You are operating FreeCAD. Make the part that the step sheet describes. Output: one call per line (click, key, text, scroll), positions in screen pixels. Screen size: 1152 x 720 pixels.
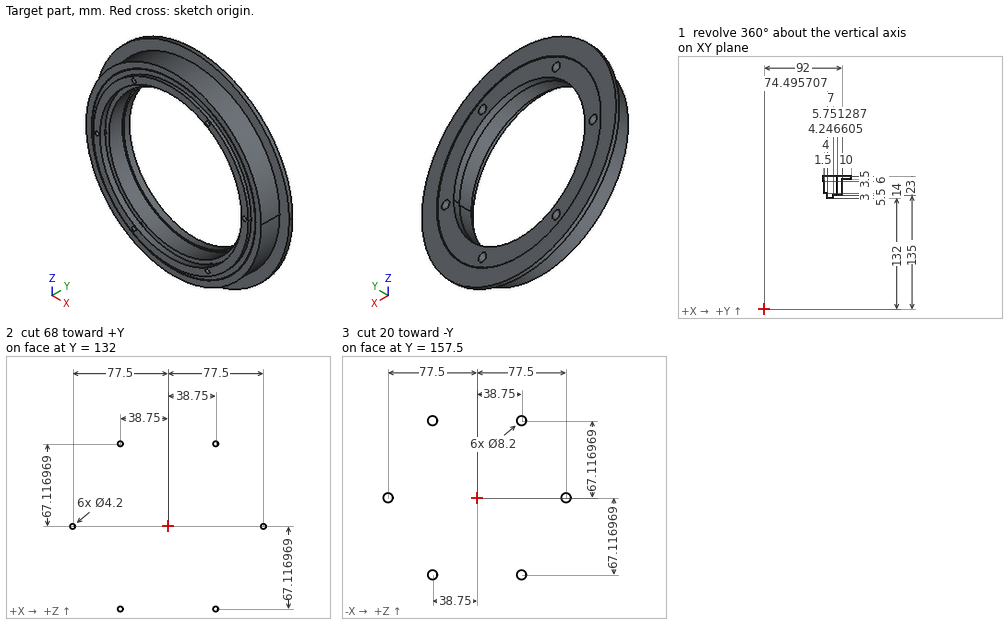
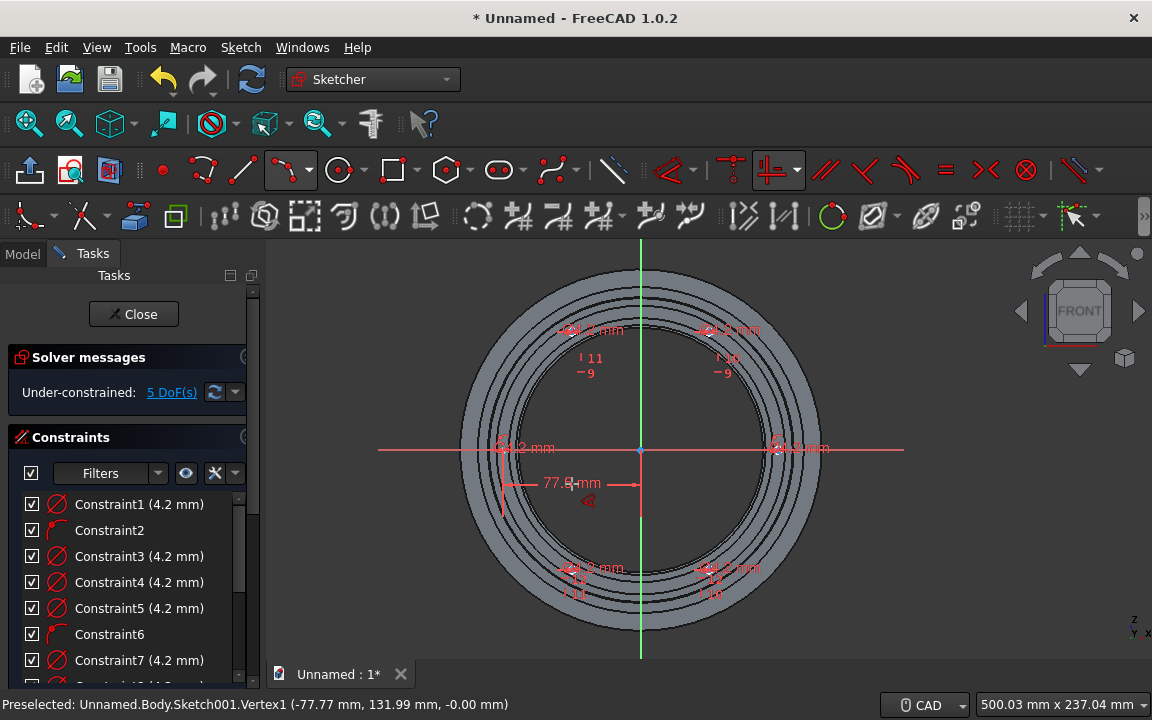
click(778, 450)
click(709, 484)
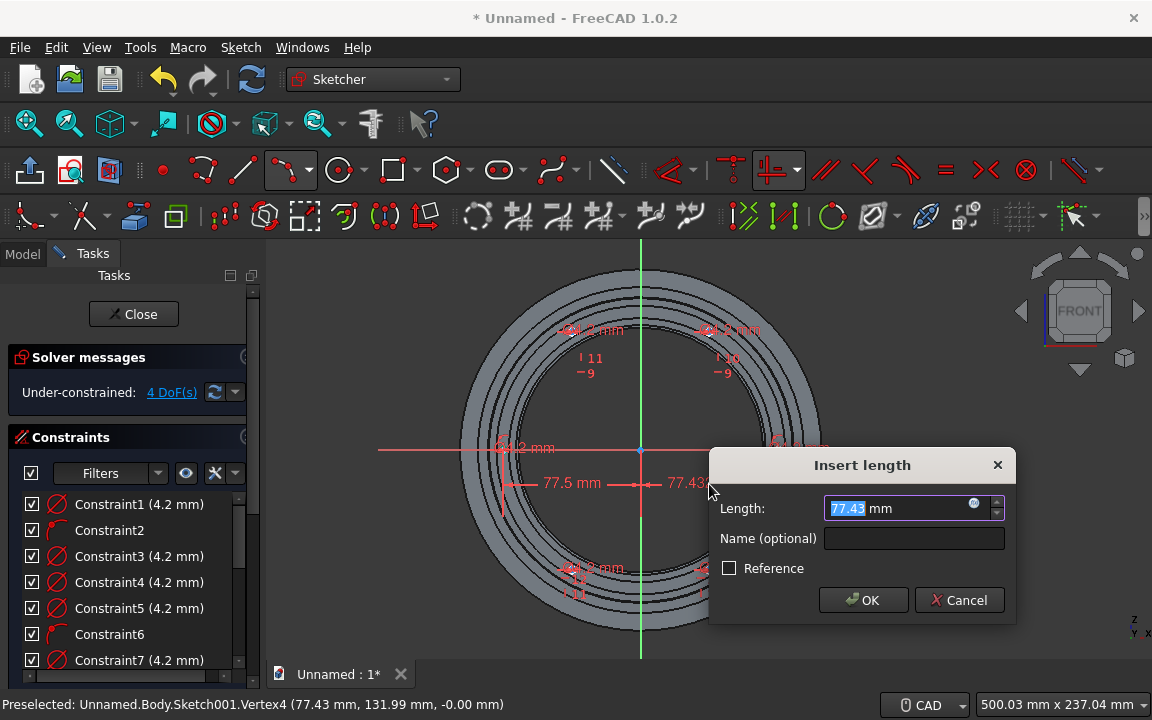
text(77.5)
key(Return)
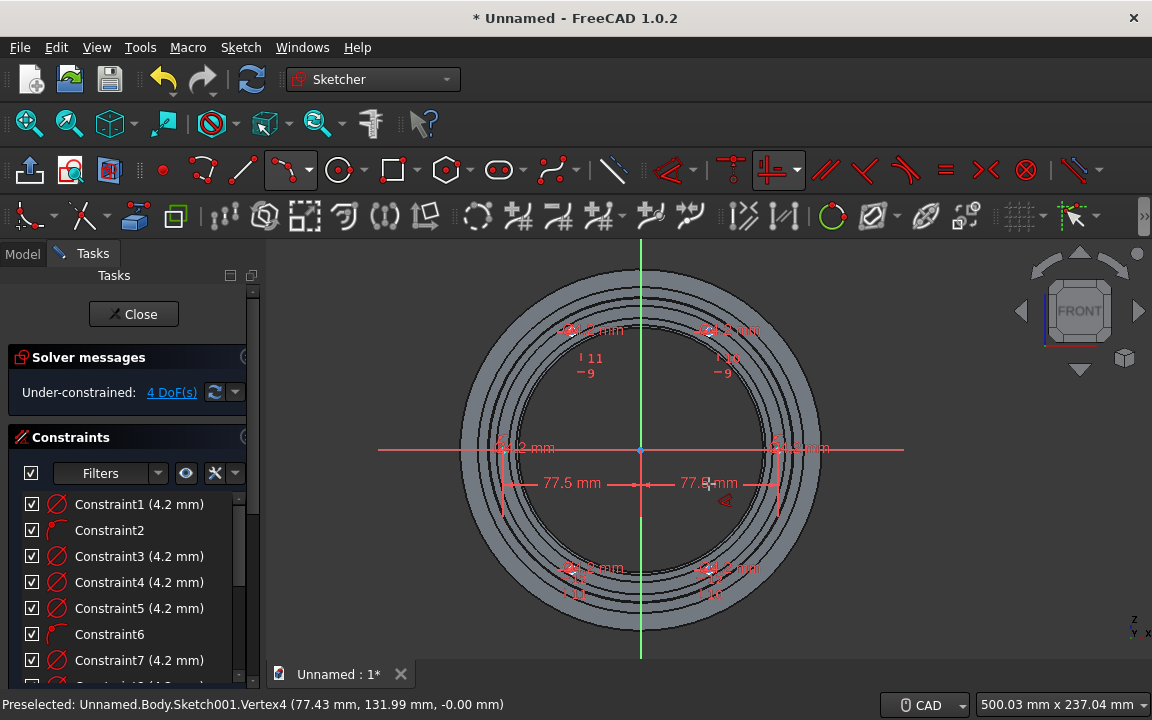
click(572, 332)
click(606, 298)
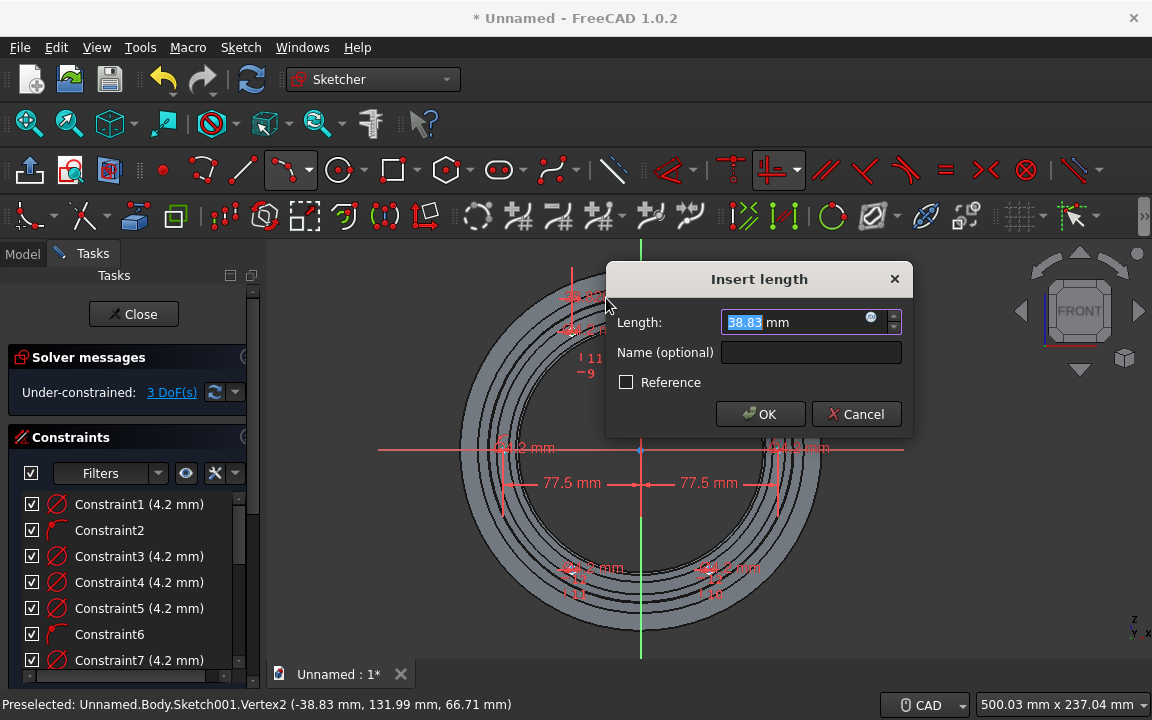
text(38.75)
key(Return)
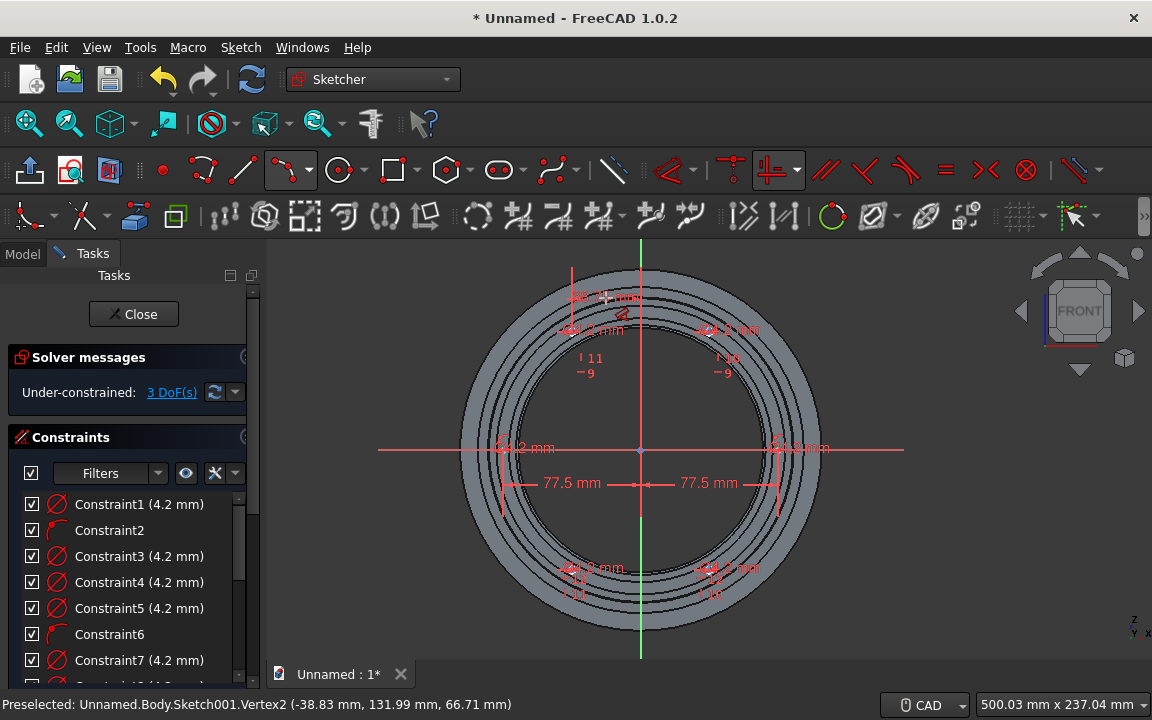
click(709, 332)
click(691, 298)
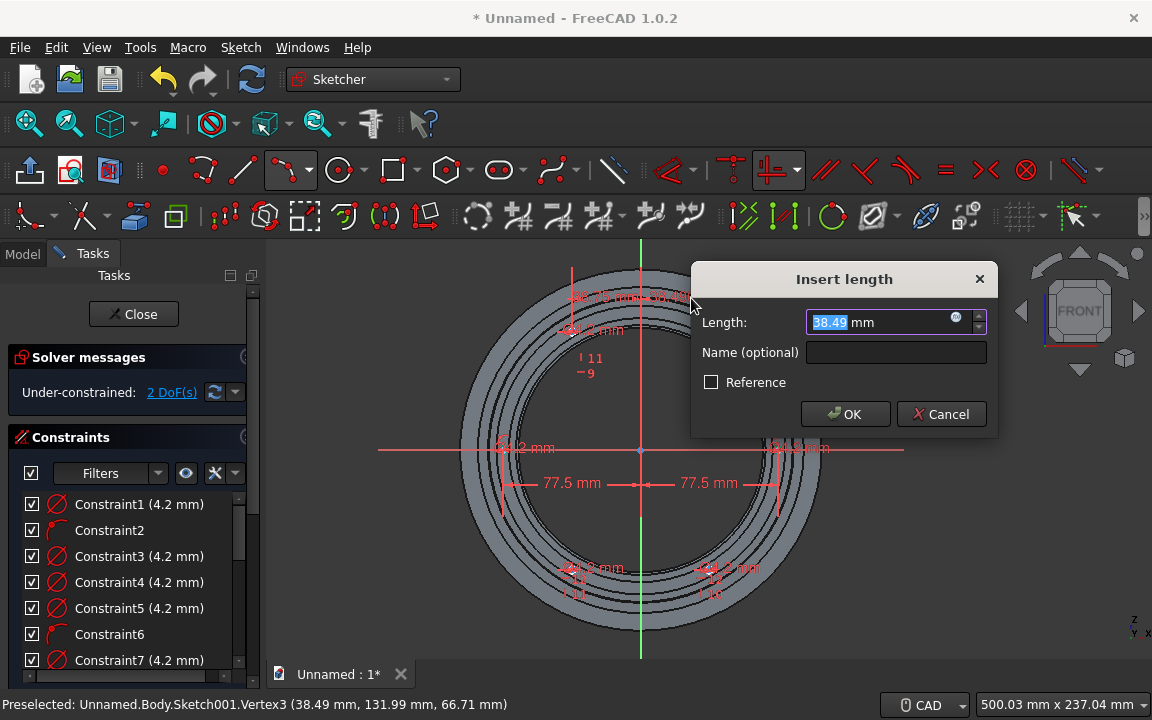
text(38.75)
key(Return)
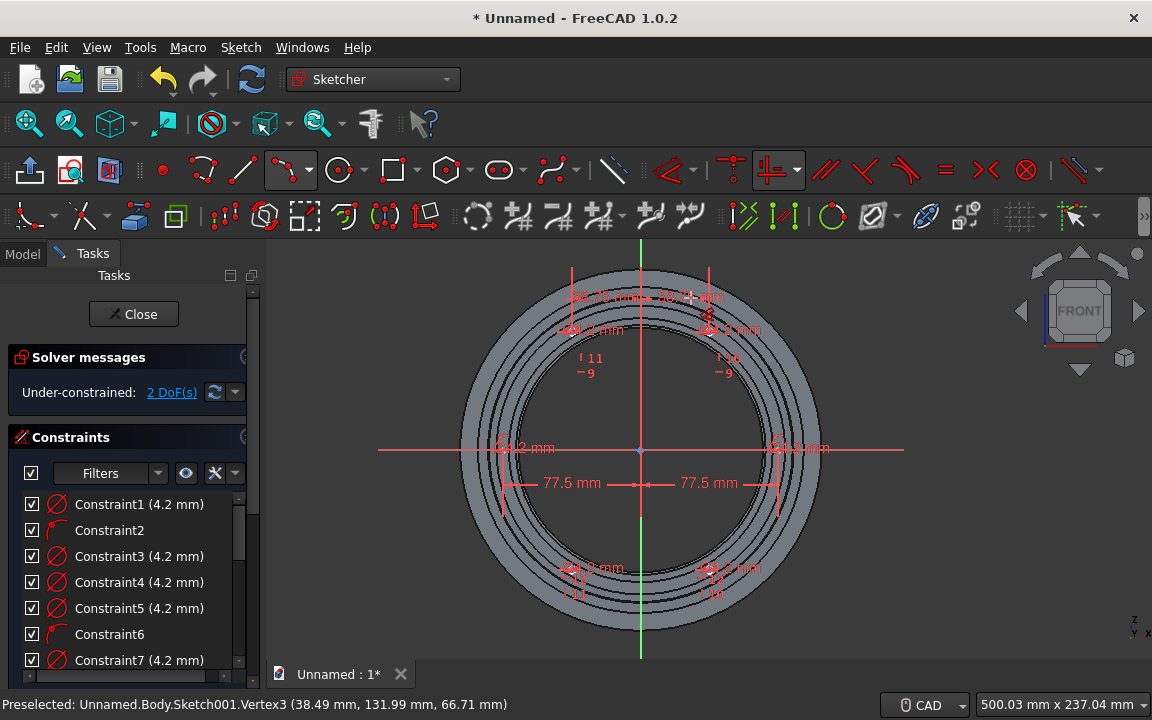
click(572, 332)
click(538, 391)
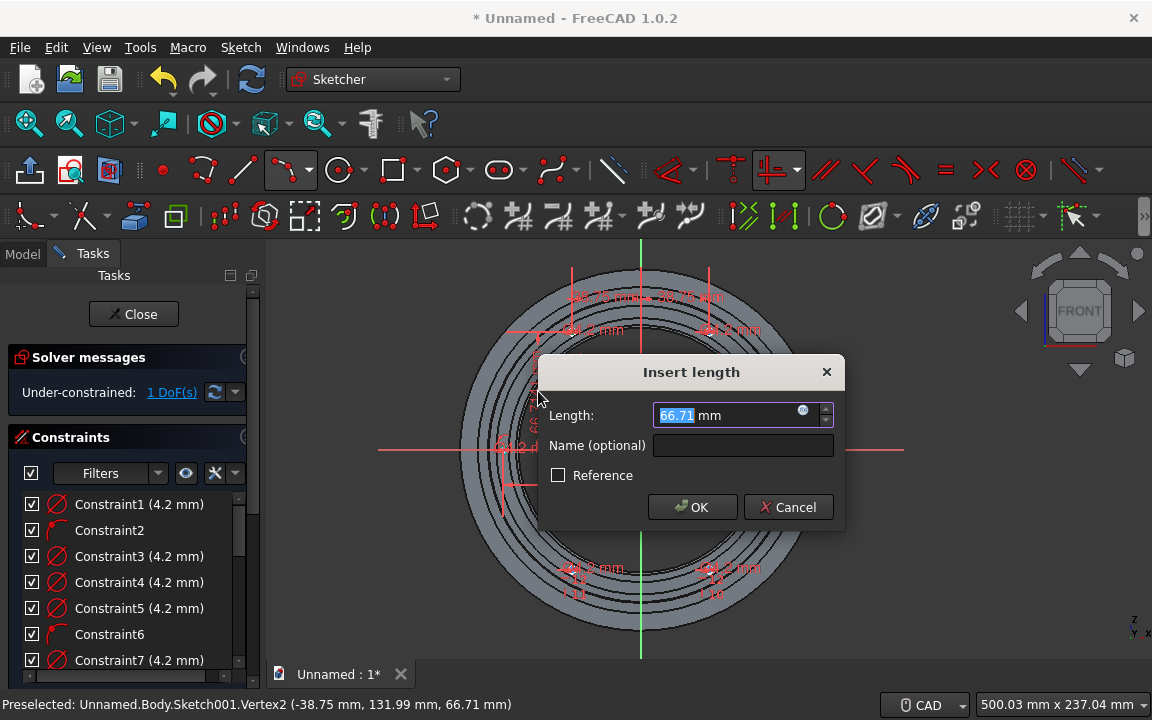
text(67.116969)
key(Return)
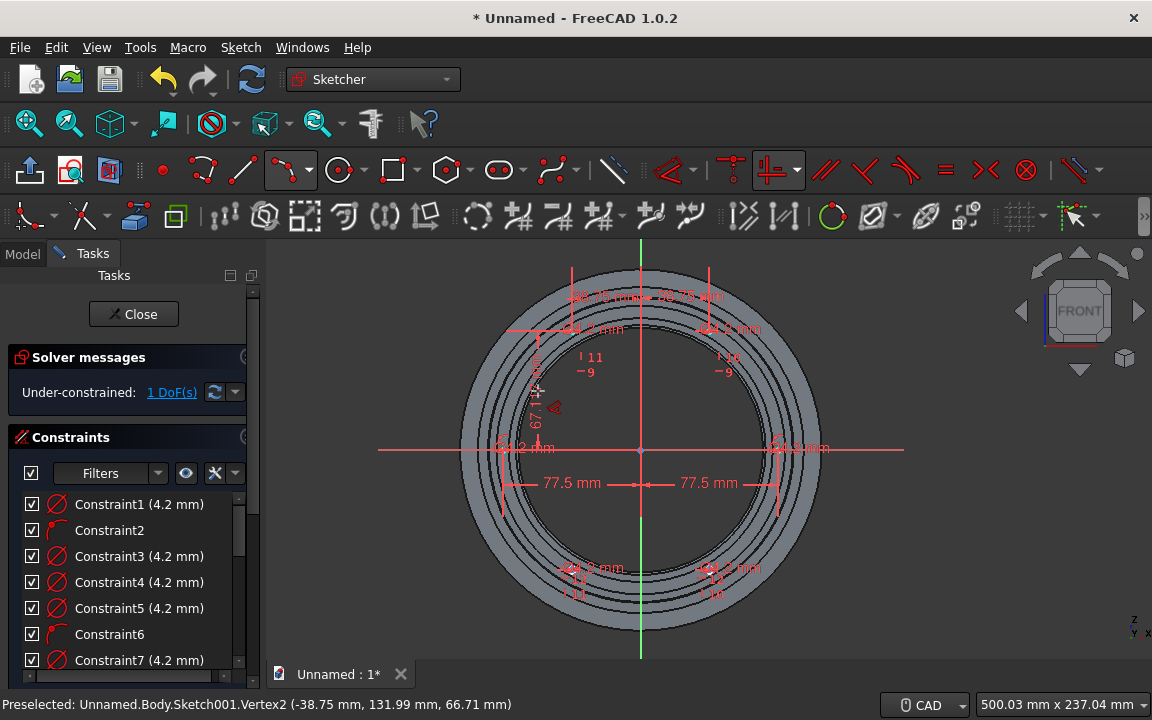
click(709, 570)
click(743, 510)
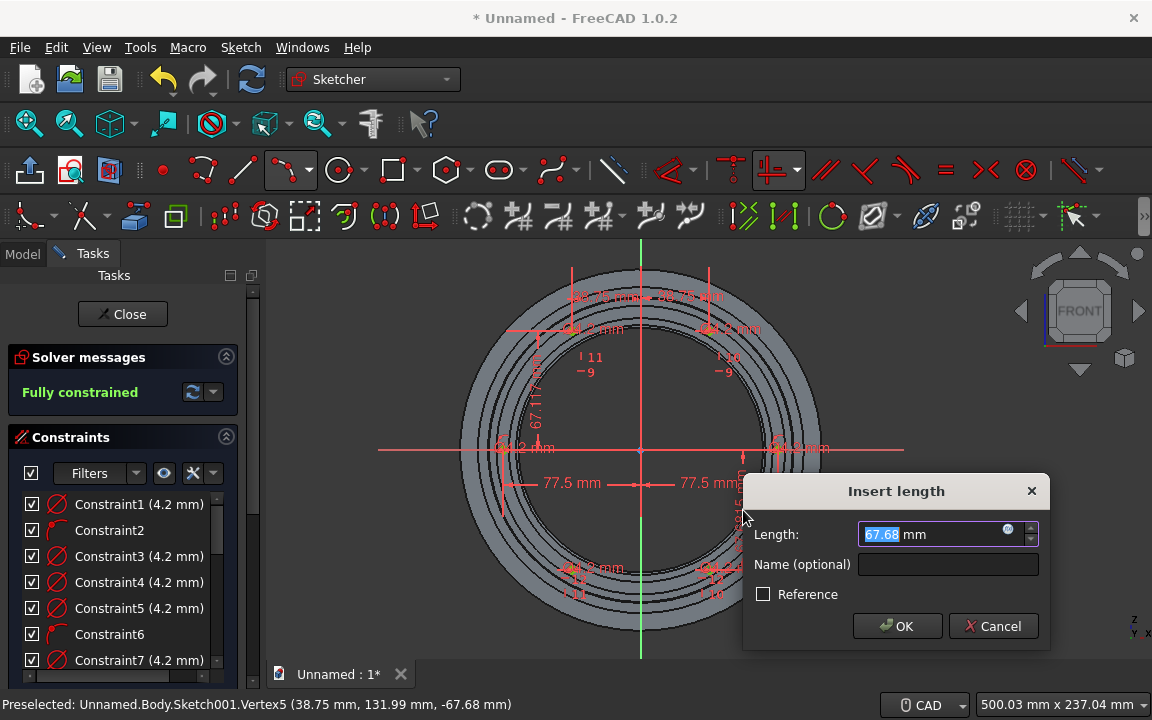
text(67.116969)
key(Return)
key(Escape)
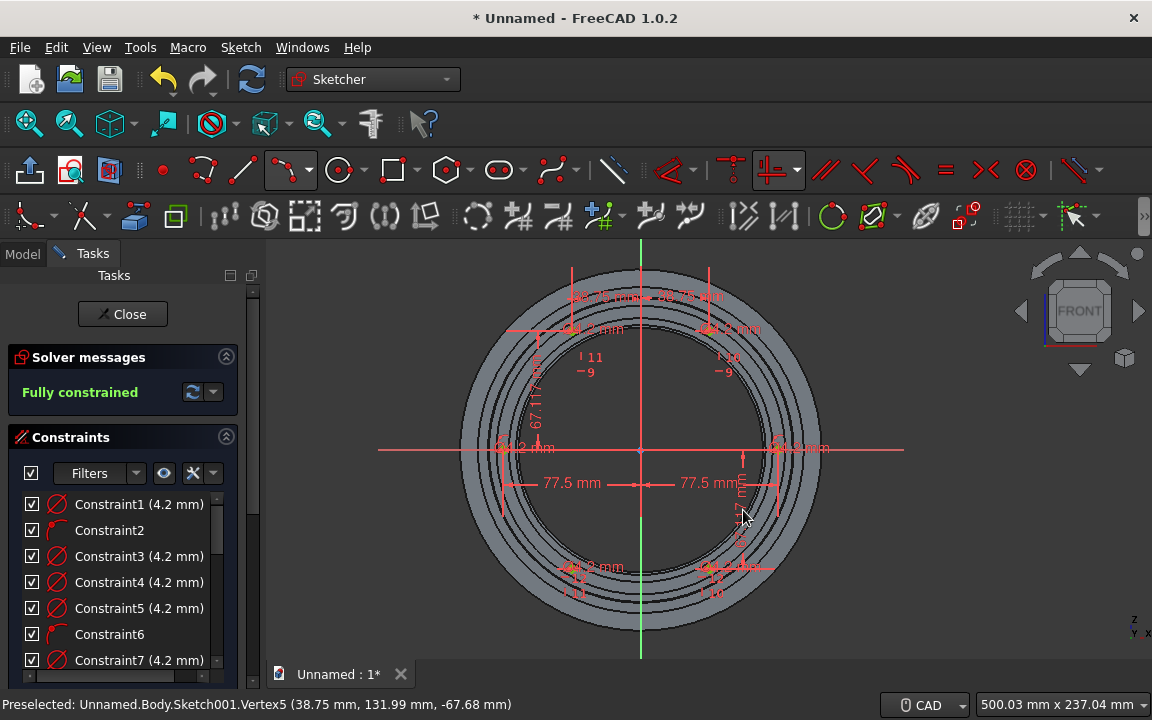
click(123, 314)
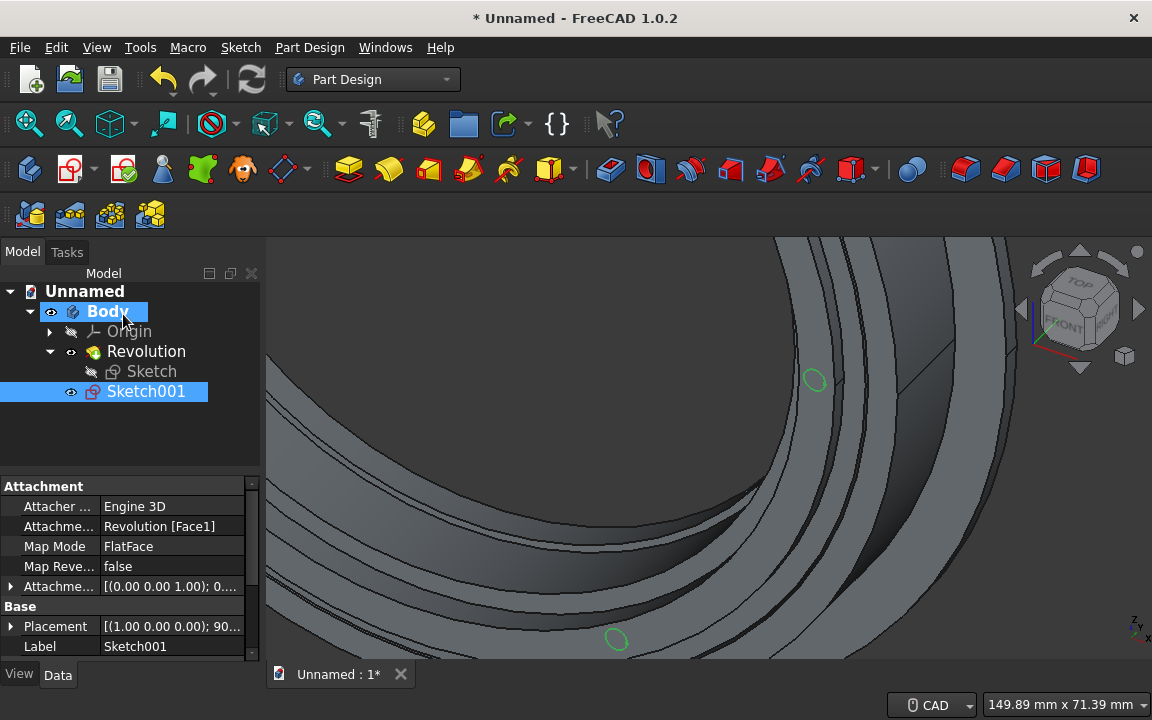
click(612, 170)